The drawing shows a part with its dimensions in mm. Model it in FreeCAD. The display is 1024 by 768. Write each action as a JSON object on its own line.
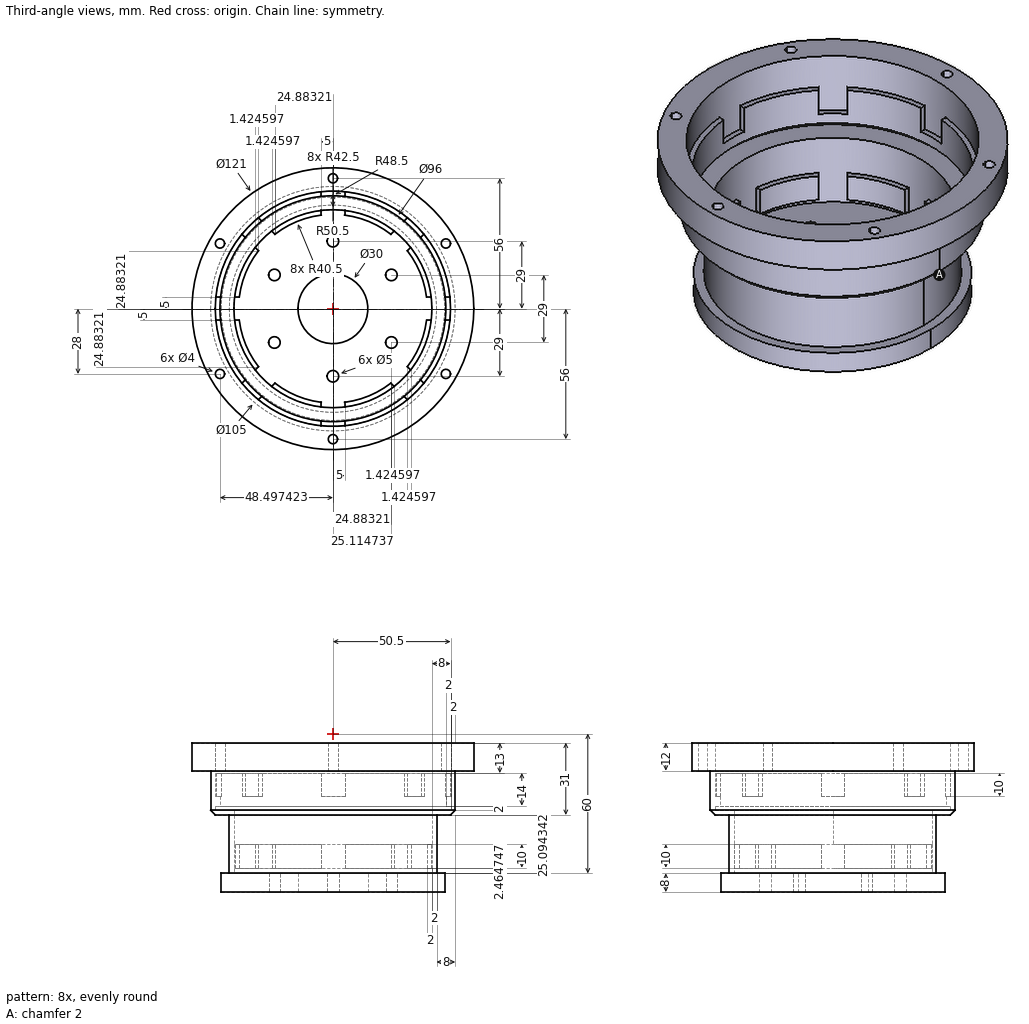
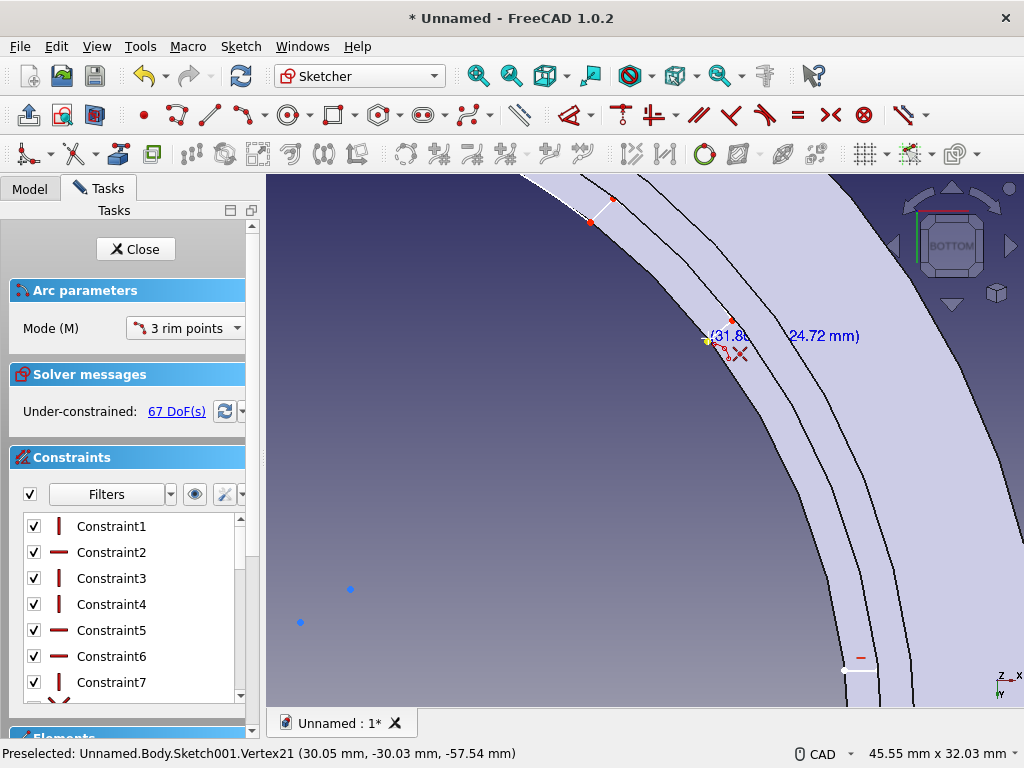
{"action": "left_click", "coordinate": [708, 341]}
{"action": "left_click", "coordinate": [844, 671]}
{"action": "left_click", "coordinate": [799, 494]}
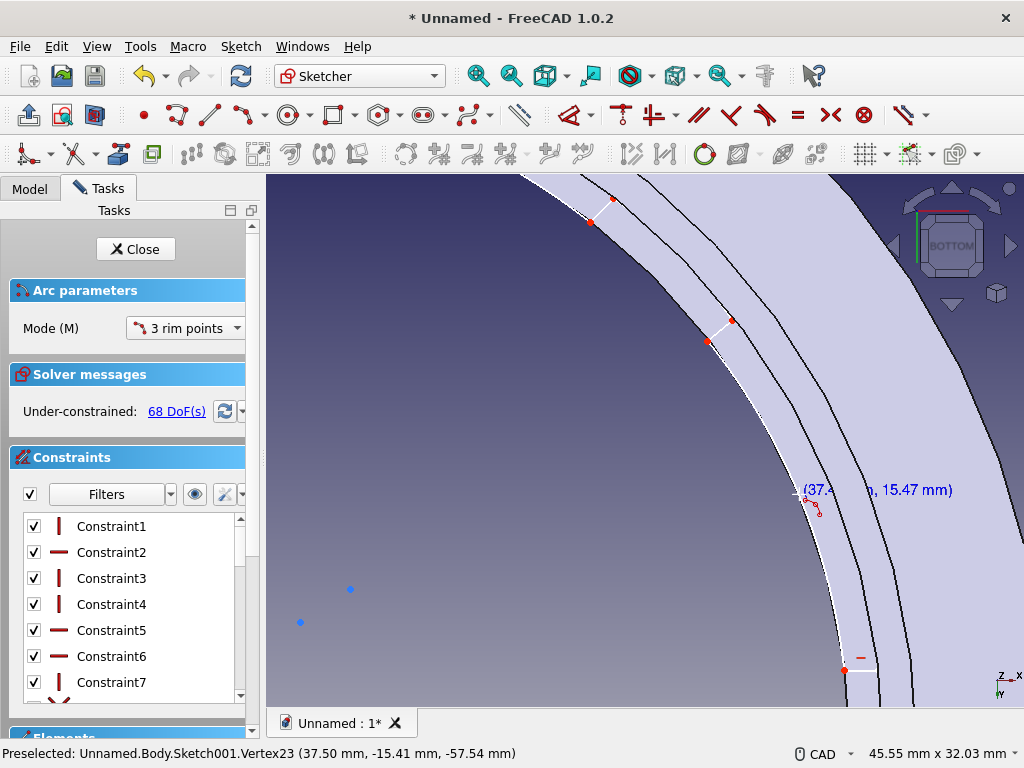
{"action": "scroll", "coordinate": [708, 338], "scroll_direction": "down", "scroll_amount": 7}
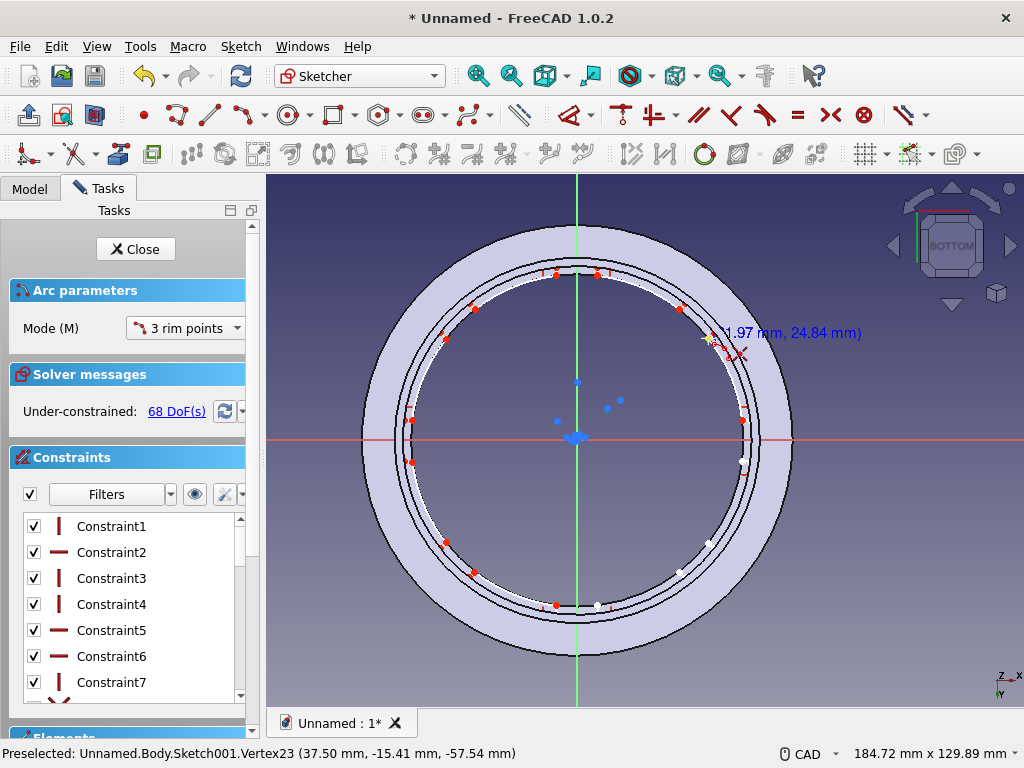
{"action": "scroll", "coordinate": [750, 420], "scroll_direction": "up", "scroll_amount": 7}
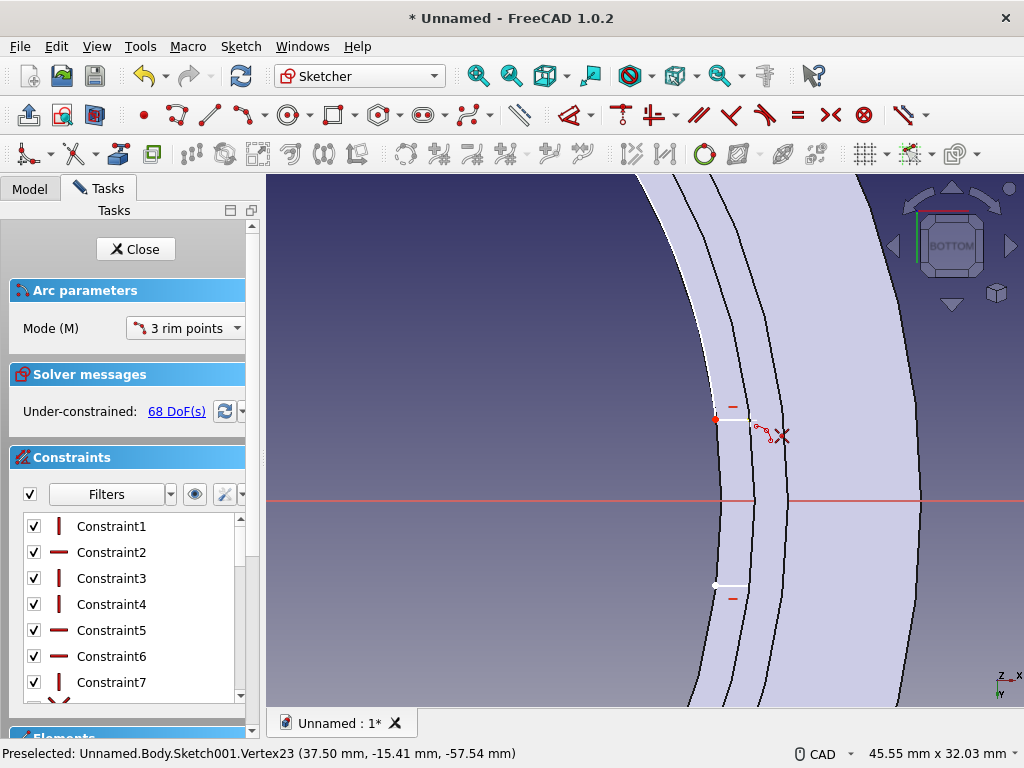
{"action": "left_click", "coordinate": [750, 420]}
{"action": "left_click", "coordinate": [750, 586]}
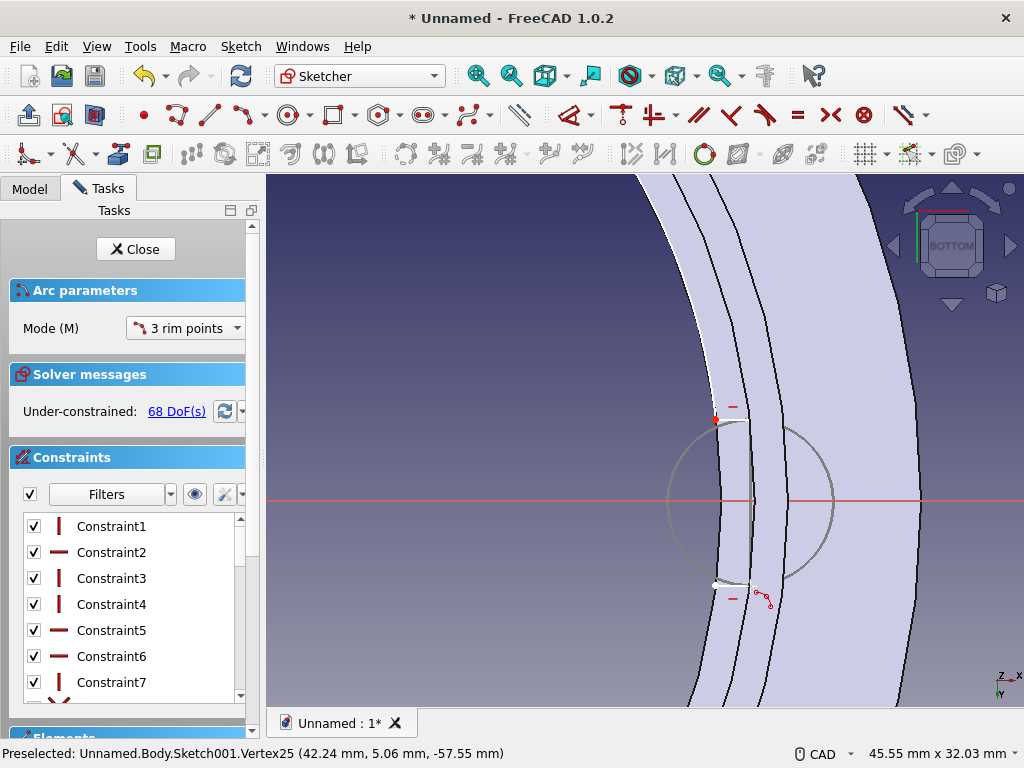
{"action": "scroll", "coordinate": [755, 518], "scroll_direction": "up", "scroll_amount": 7}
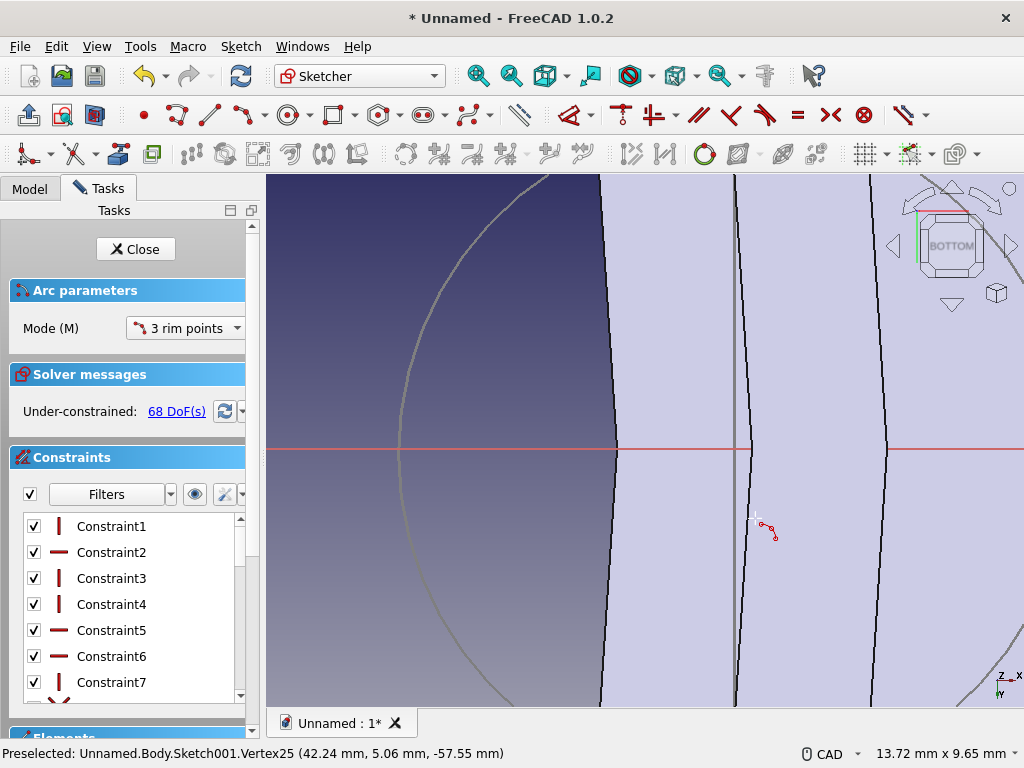
{"action": "left_click", "coordinate": [751, 516]}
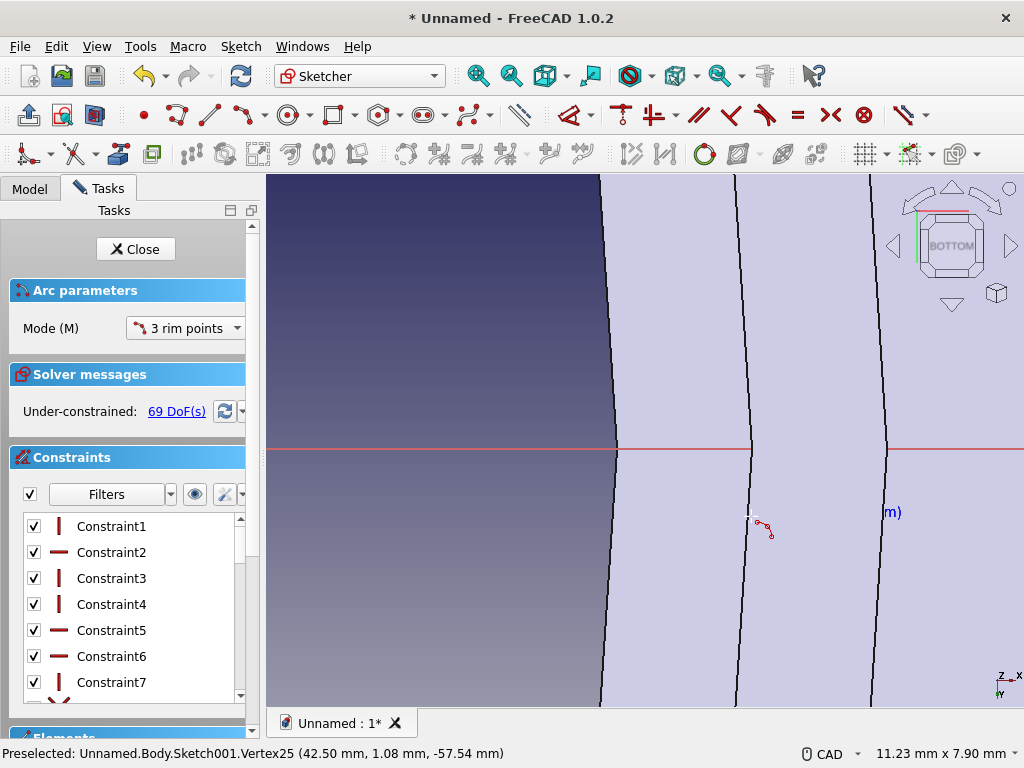
{"action": "scroll", "coordinate": [751, 440], "scroll_direction": "down", "scroll_amount": 14}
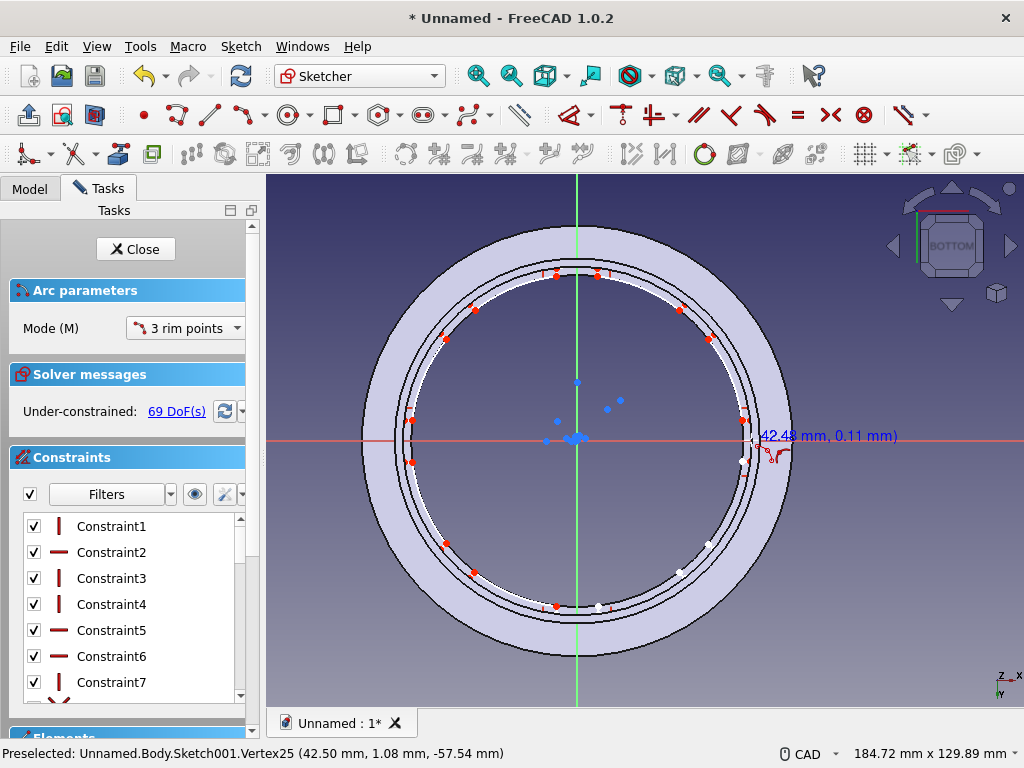
{"action": "scroll", "coordinate": [742, 462], "scroll_direction": "up", "scroll_amount": 7}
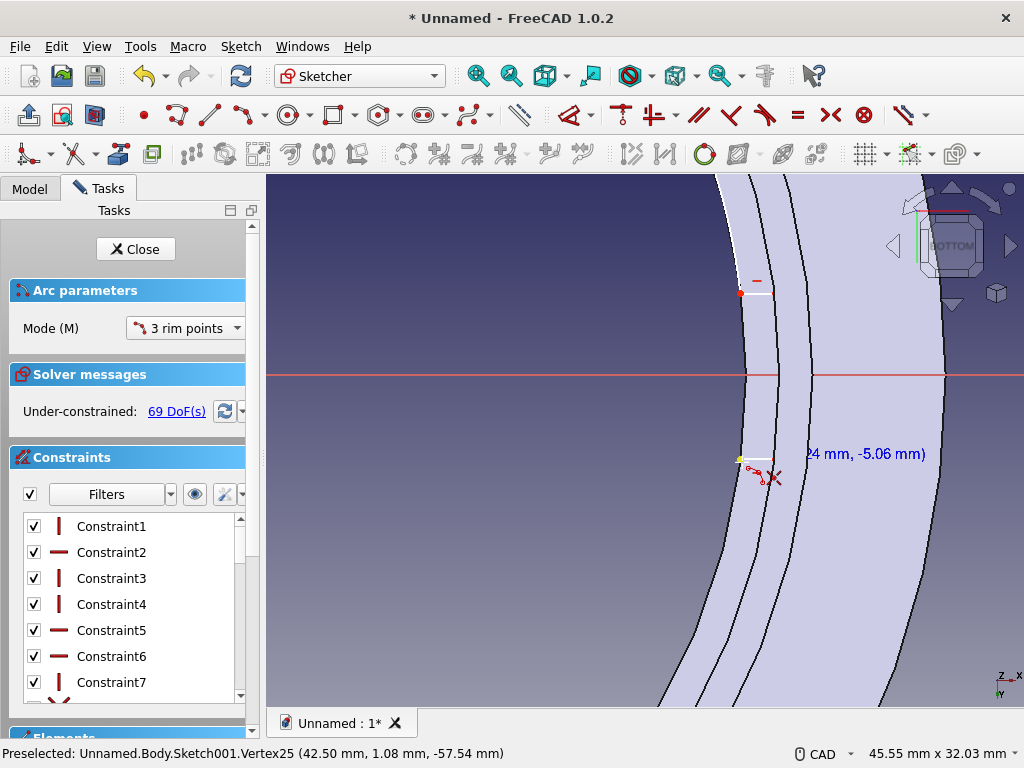
{"action": "left_click", "coordinate": [740, 459]}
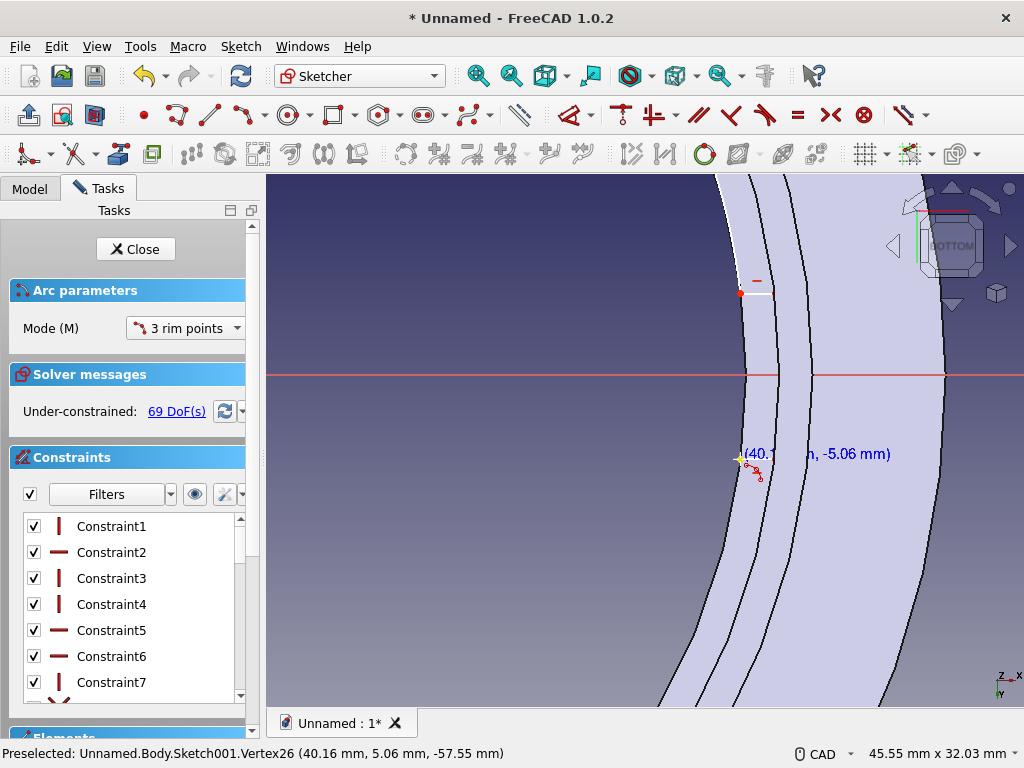
{"action": "scroll", "coordinate": [742, 462], "scroll_direction": "down", "scroll_amount": 7}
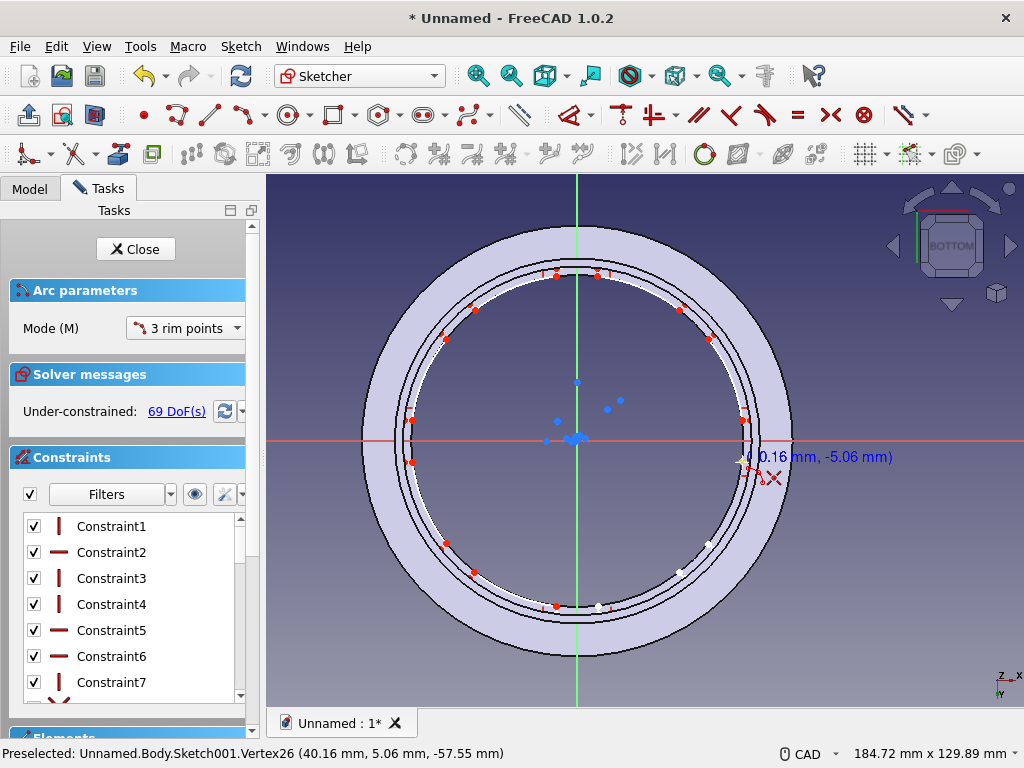
{"action": "scroll", "coordinate": [708, 543], "scroll_direction": "up", "scroll_amount": 7}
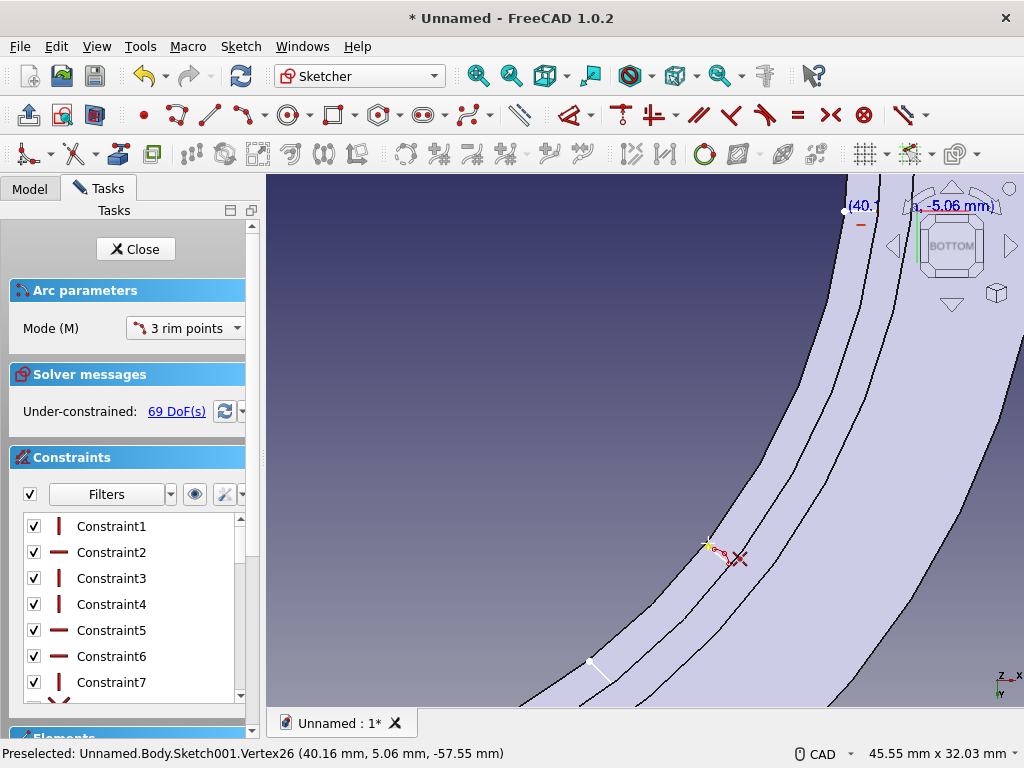
{"action": "left_click", "coordinate": [708, 547]}
{"action": "left_click", "coordinate": [799, 385]}